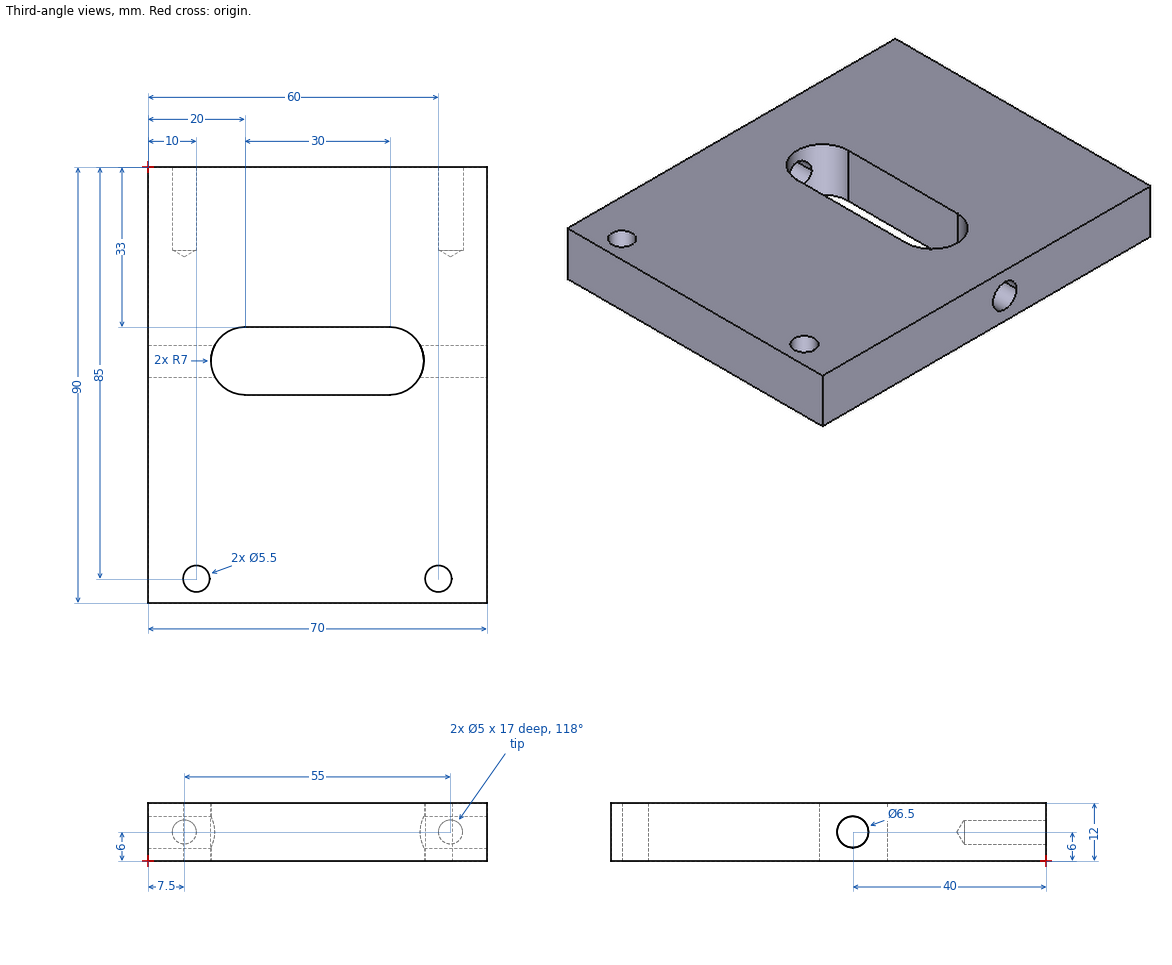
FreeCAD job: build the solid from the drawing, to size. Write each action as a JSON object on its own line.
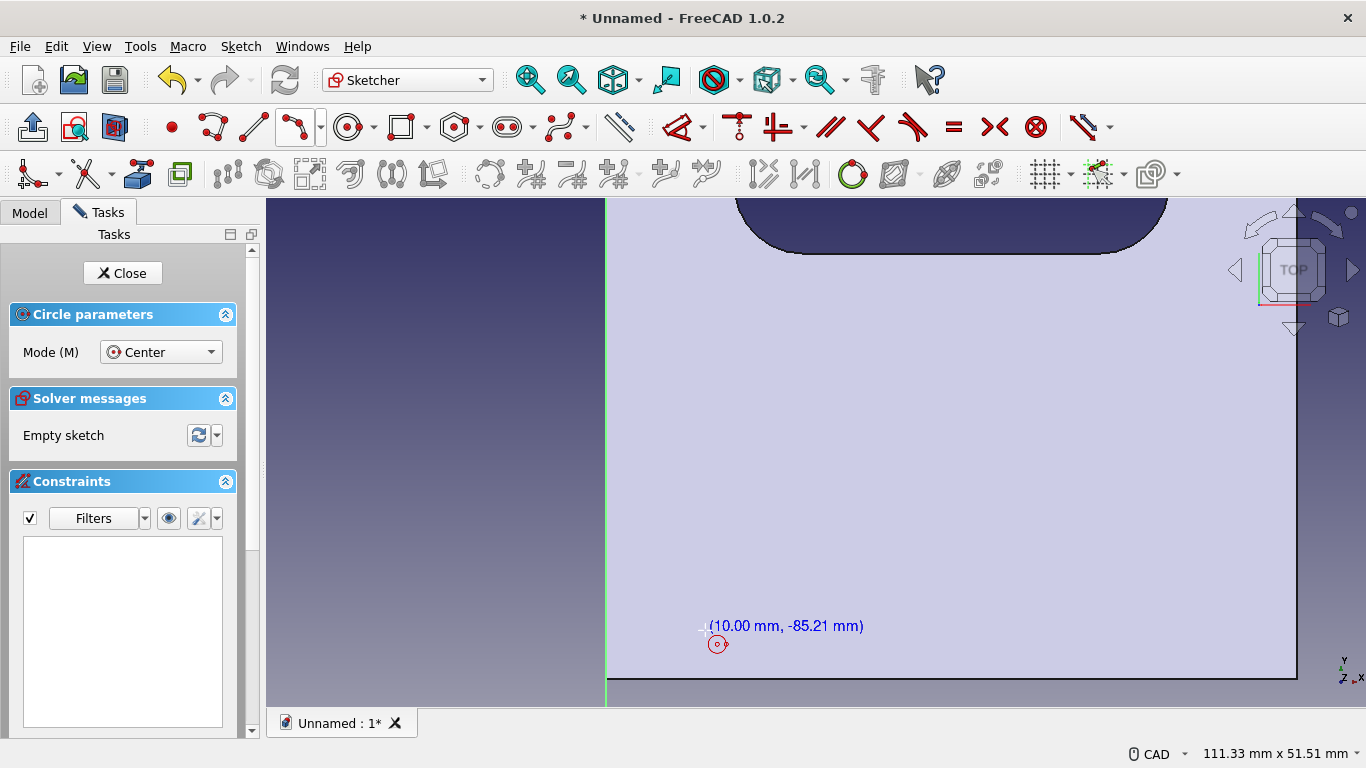
{"action": "left_click", "coordinate": [705, 629]}
{"action": "left_click", "coordinate": [724, 610]}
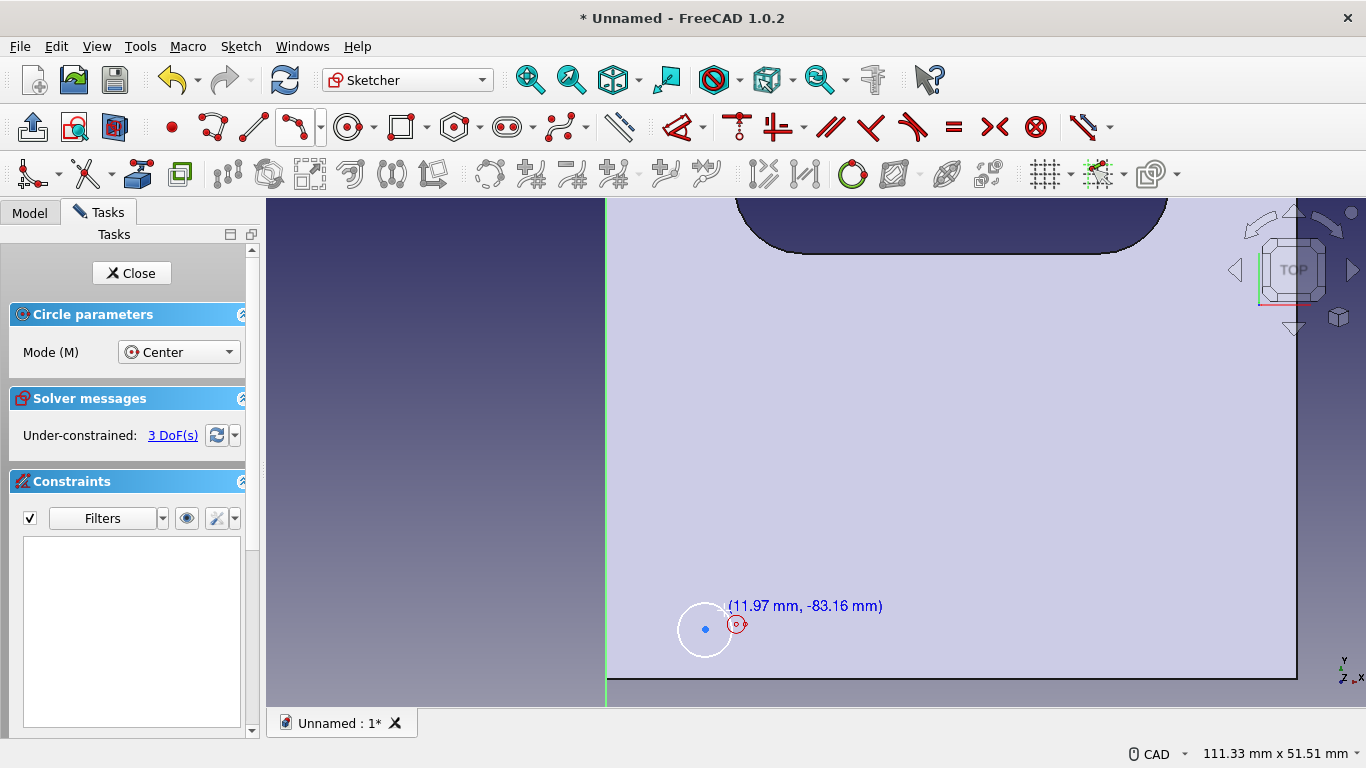
{"action": "left_click", "coordinate": [1199, 629]}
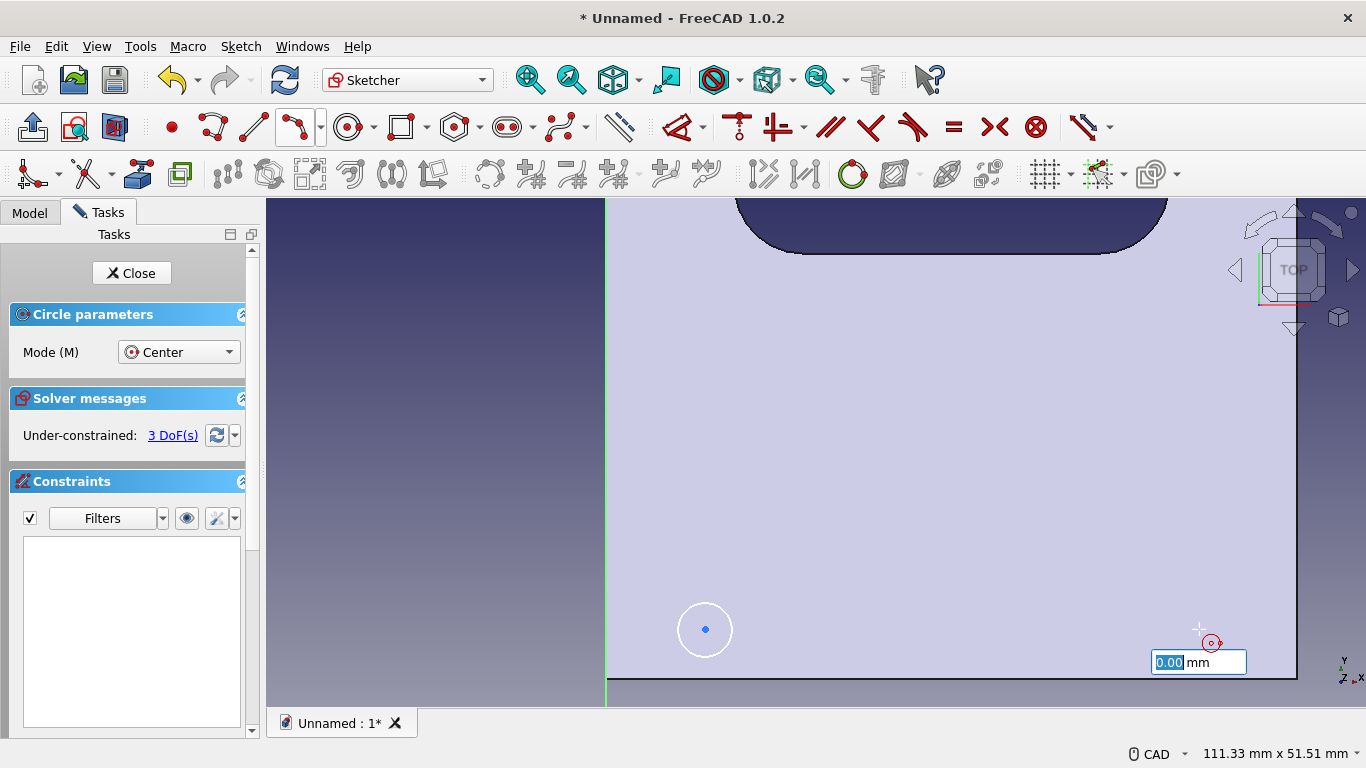
{"action": "scroll", "coordinate": [650, 586], "scroll_direction": "down", "scroll_amount": 5}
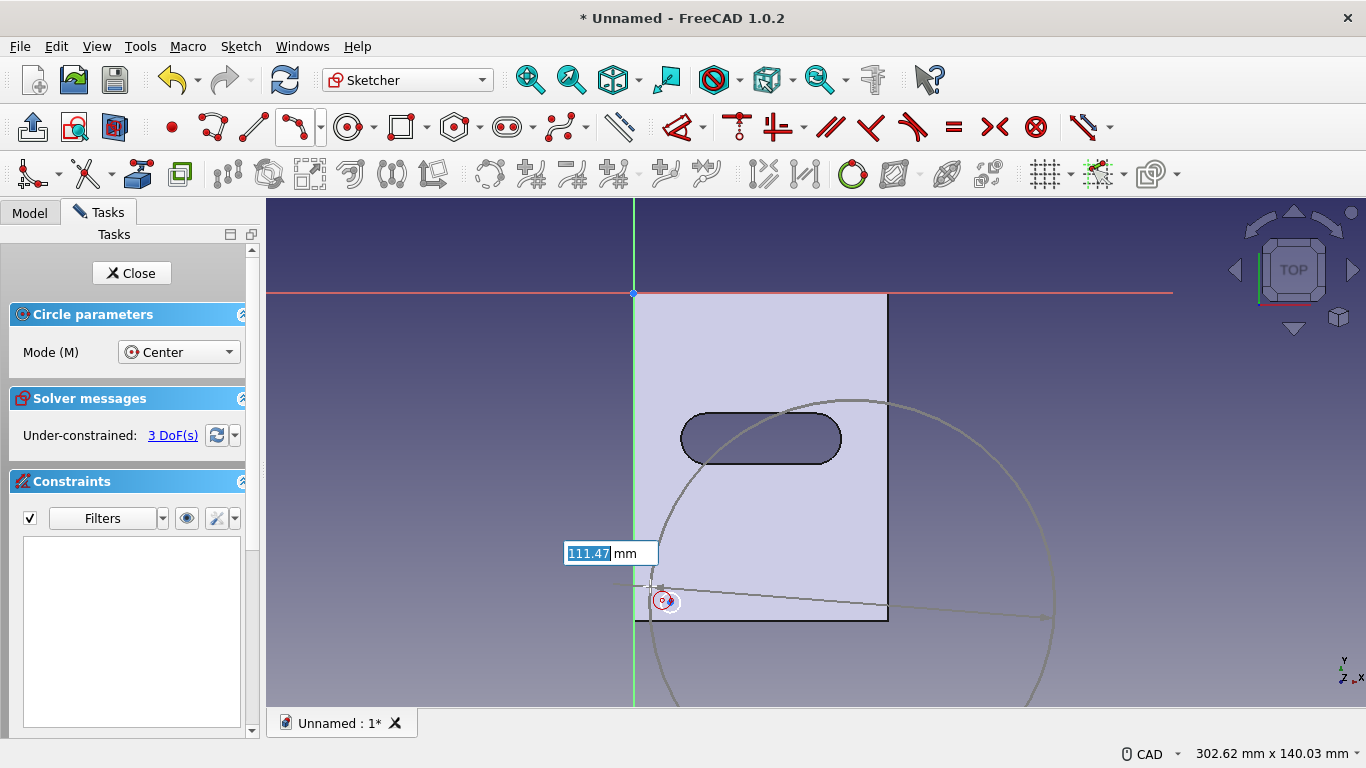
{"action": "scroll", "coordinate": [859, 595], "scroll_direction": "up", "scroll_amount": 3}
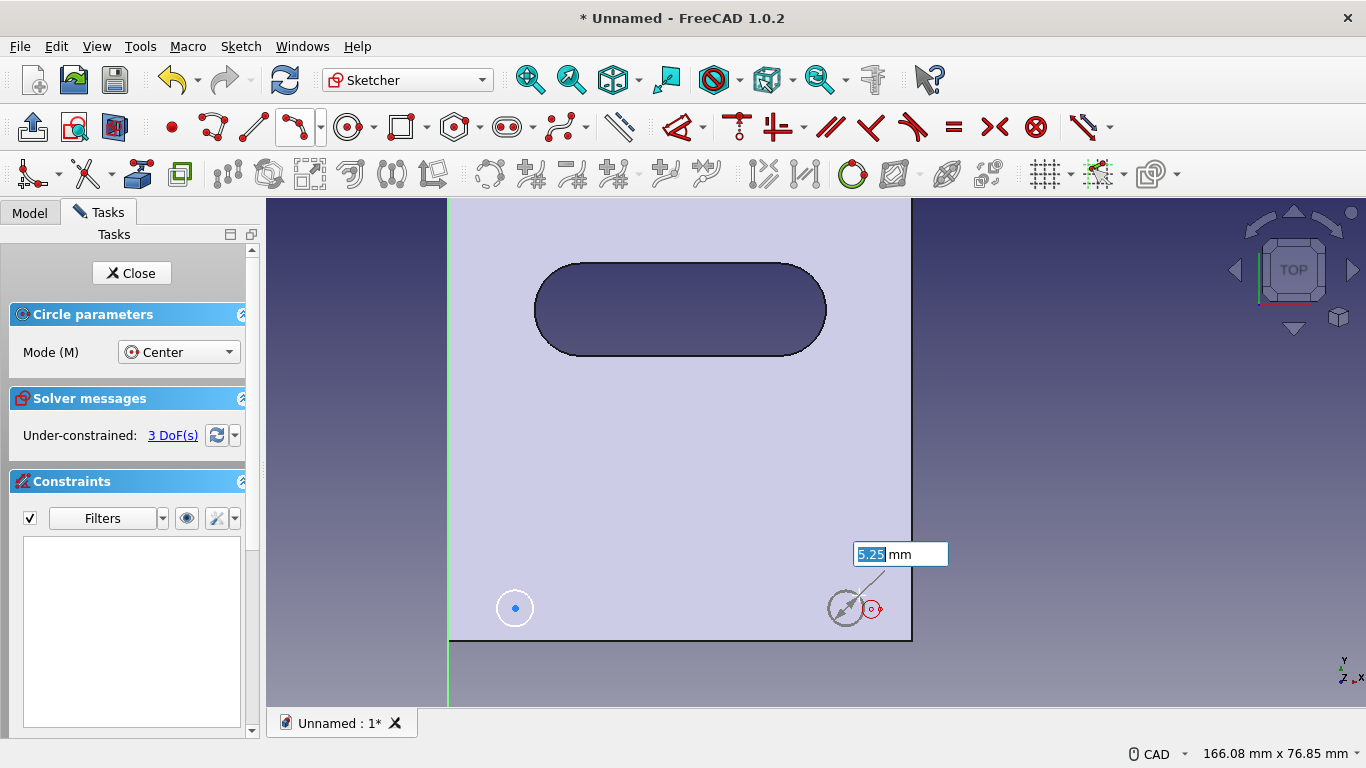
{"action": "left_click", "coordinate": [859, 595]}
{"action": "key", "text": "Escape"}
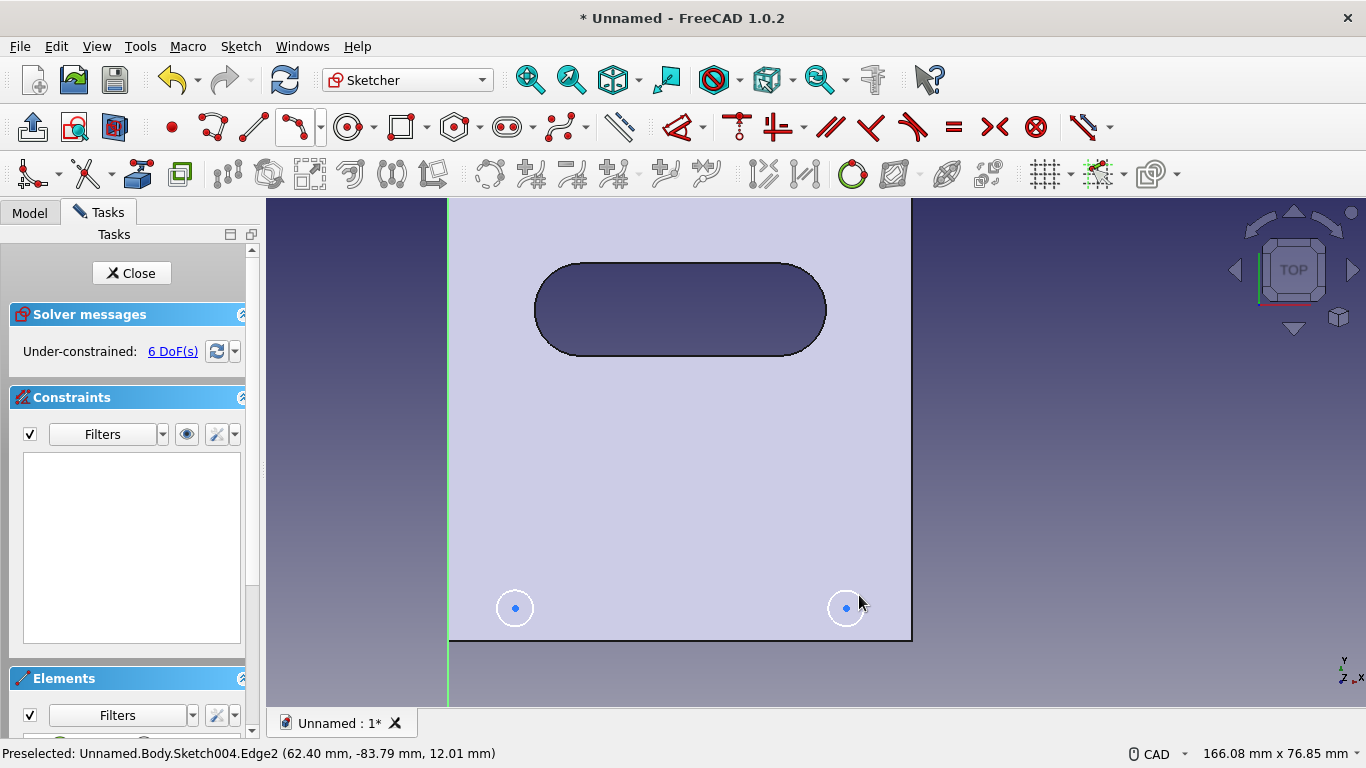
{"action": "left_click", "coordinate": [528, 596]}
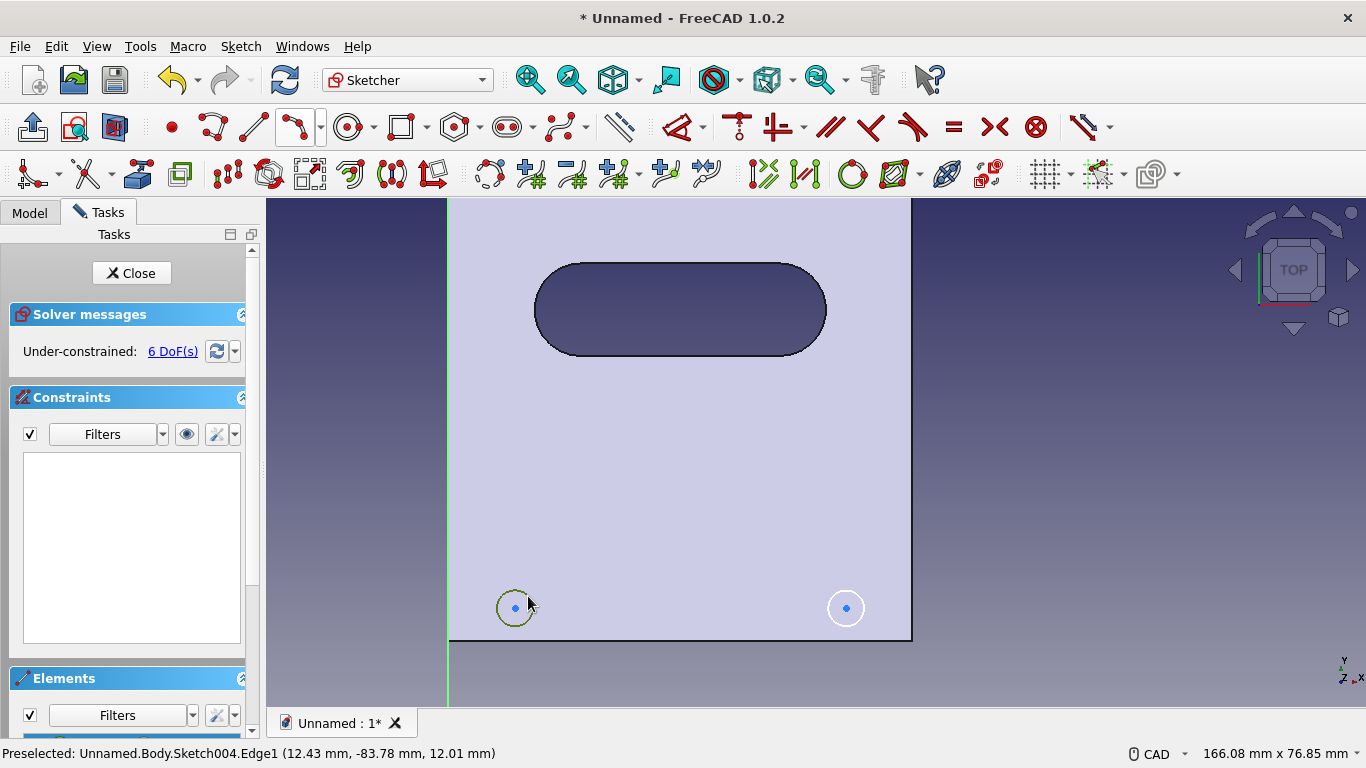
{"action": "left_click", "coordinate": [859, 596]}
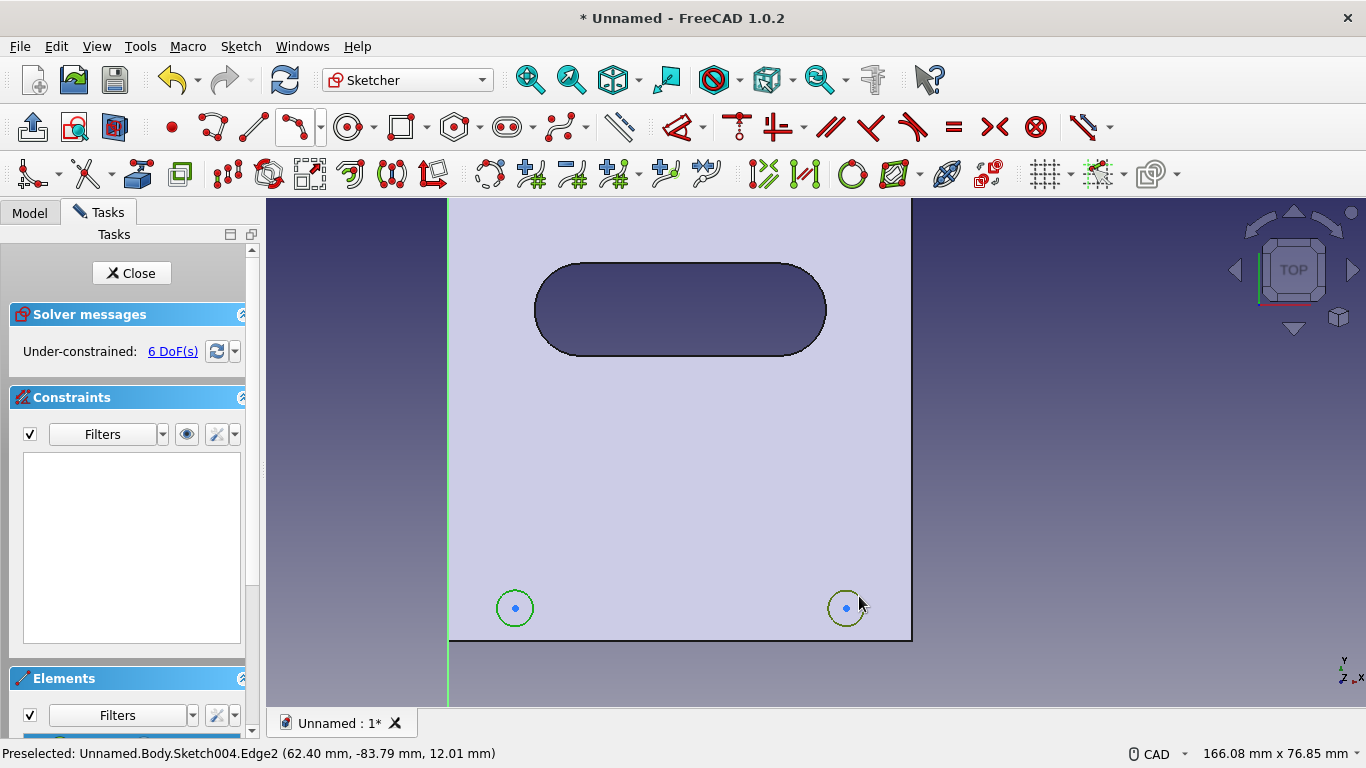
{"action": "left_click", "coordinate": [954, 128]}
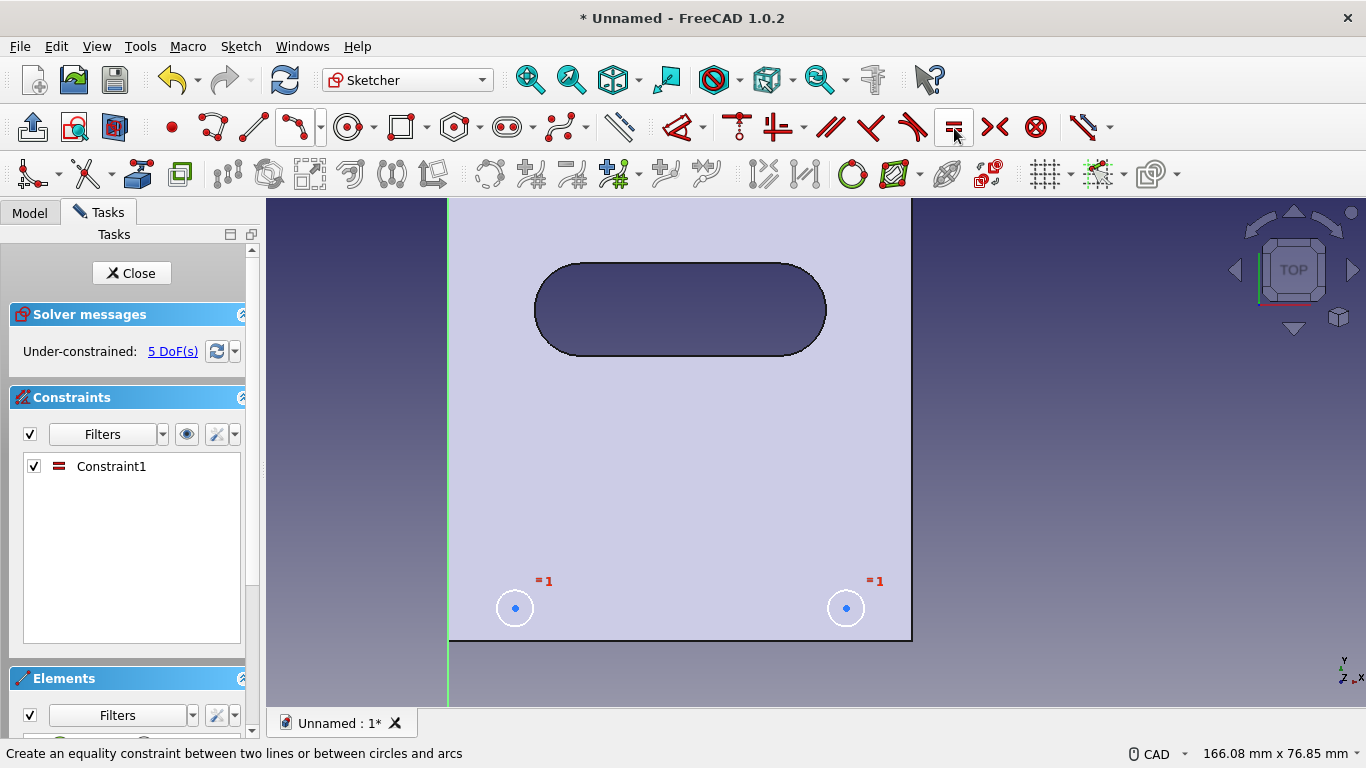
{"action": "left_click", "coordinate": [676, 128]}